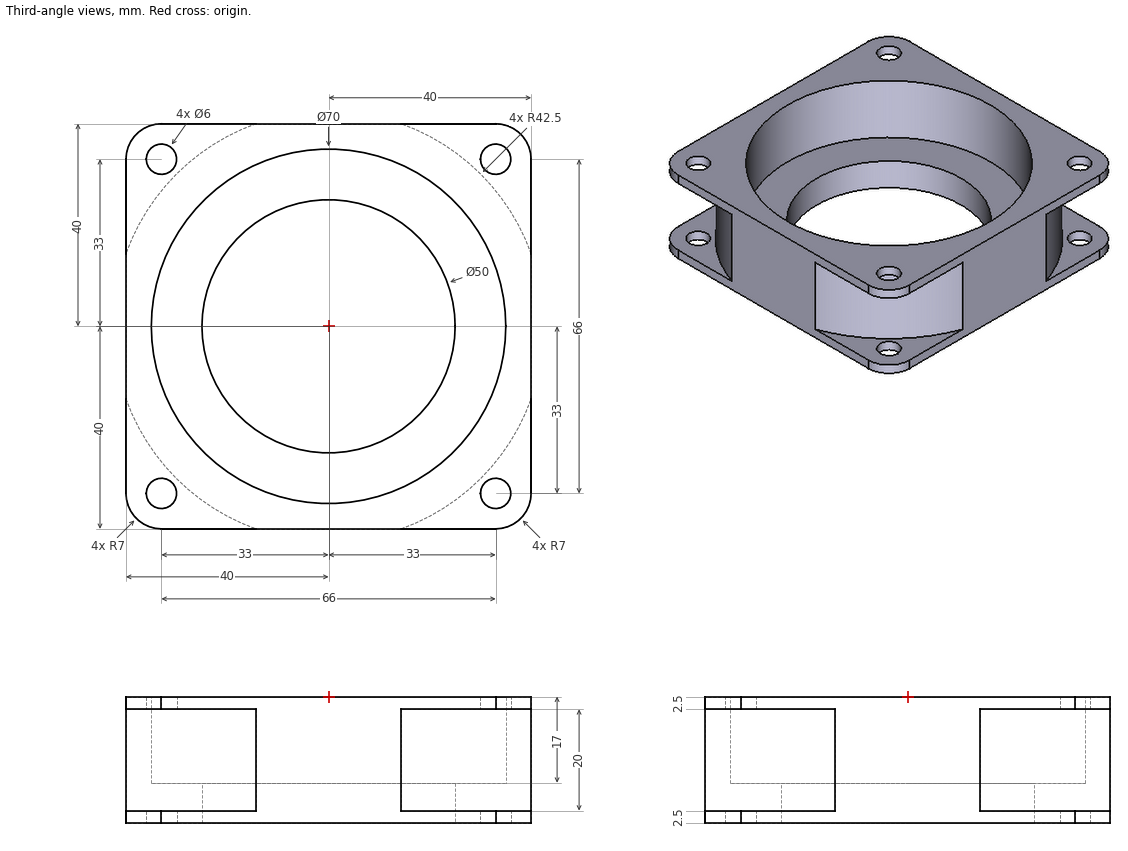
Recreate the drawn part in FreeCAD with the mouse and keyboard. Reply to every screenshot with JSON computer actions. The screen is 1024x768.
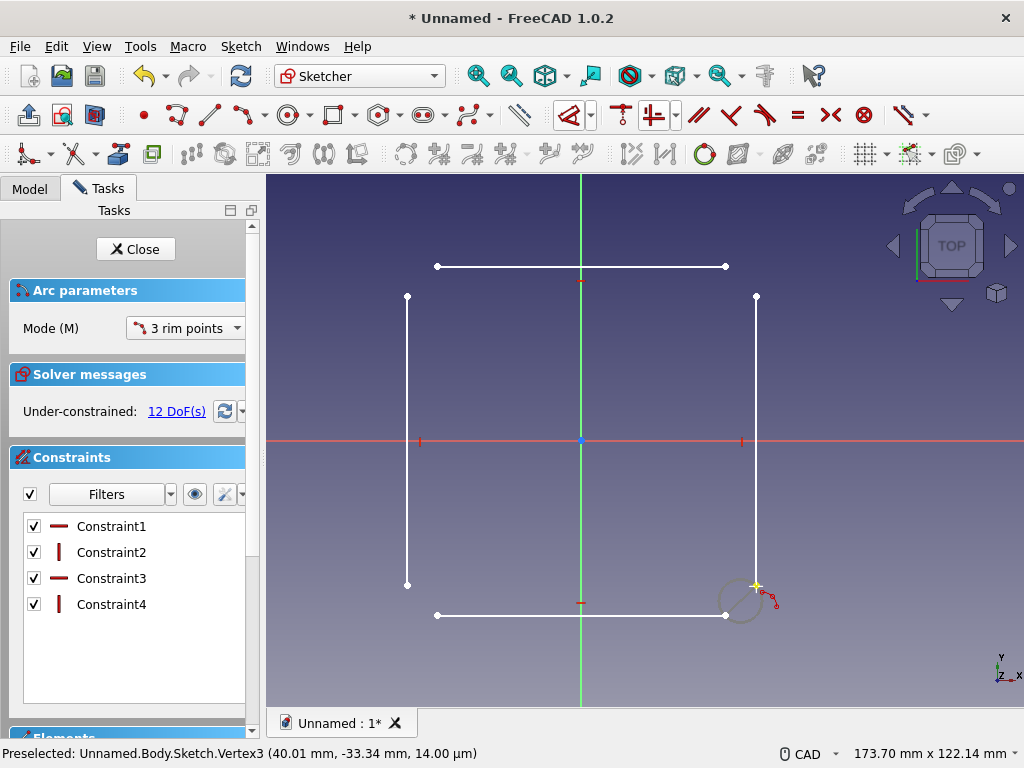
{"action": "scroll", "coordinate": [747, 606], "scroll_direction": "up", "scroll_amount": 3}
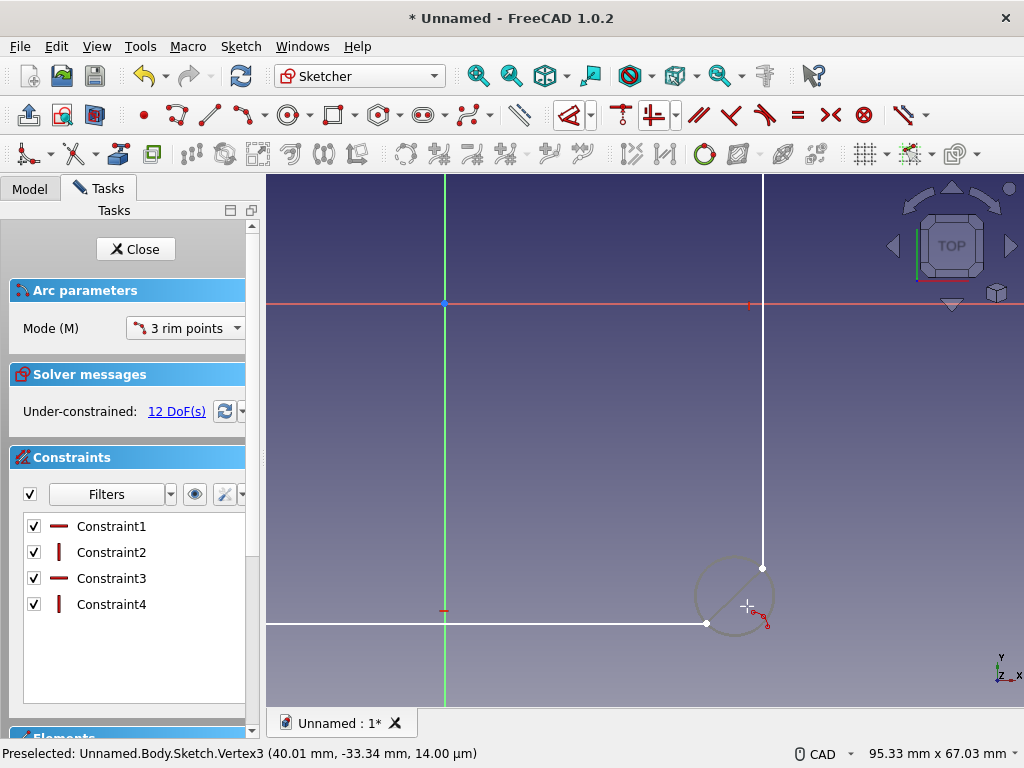
{"action": "left_click", "coordinate": [746, 606]}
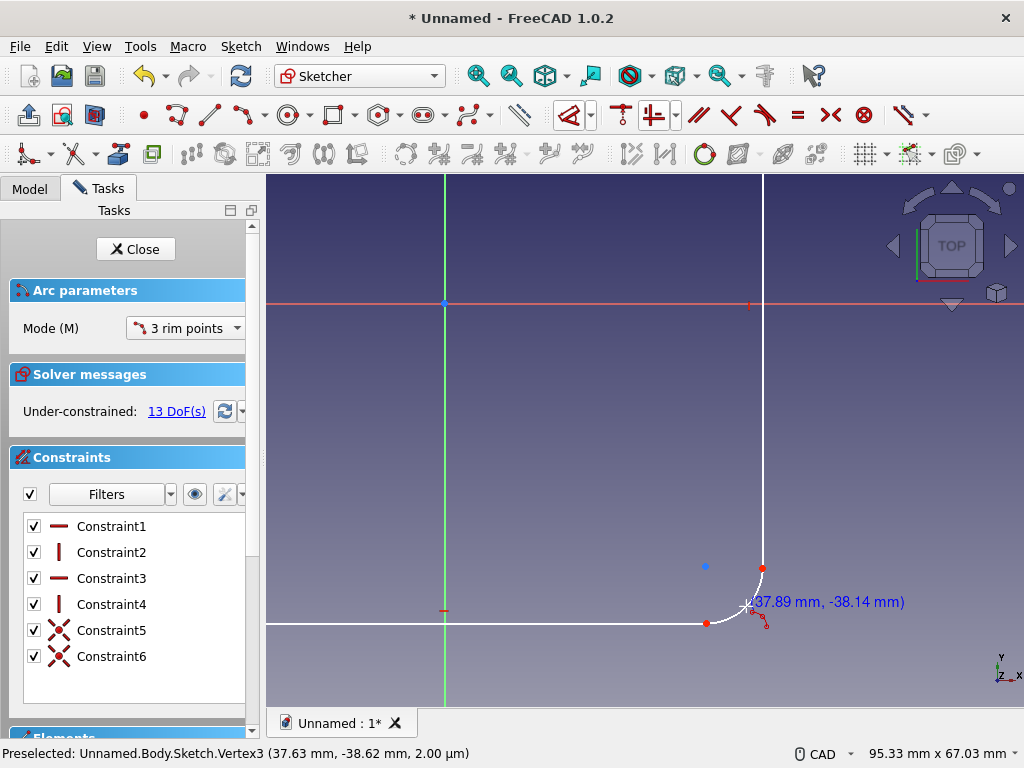
{"action": "scroll", "coordinate": [737, 607], "scroll_direction": "down", "scroll_amount": 3}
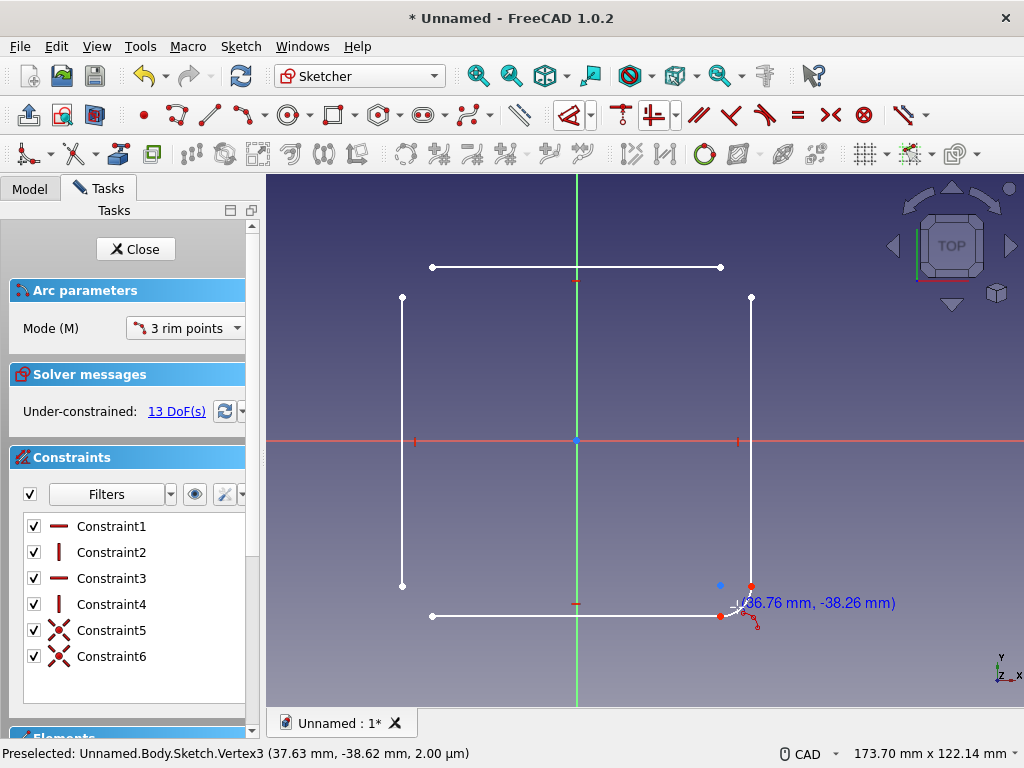
{"action": "left_click", "coordinate": [751, 297]}
{"action": "left_click", "coordinate": [720, 267]}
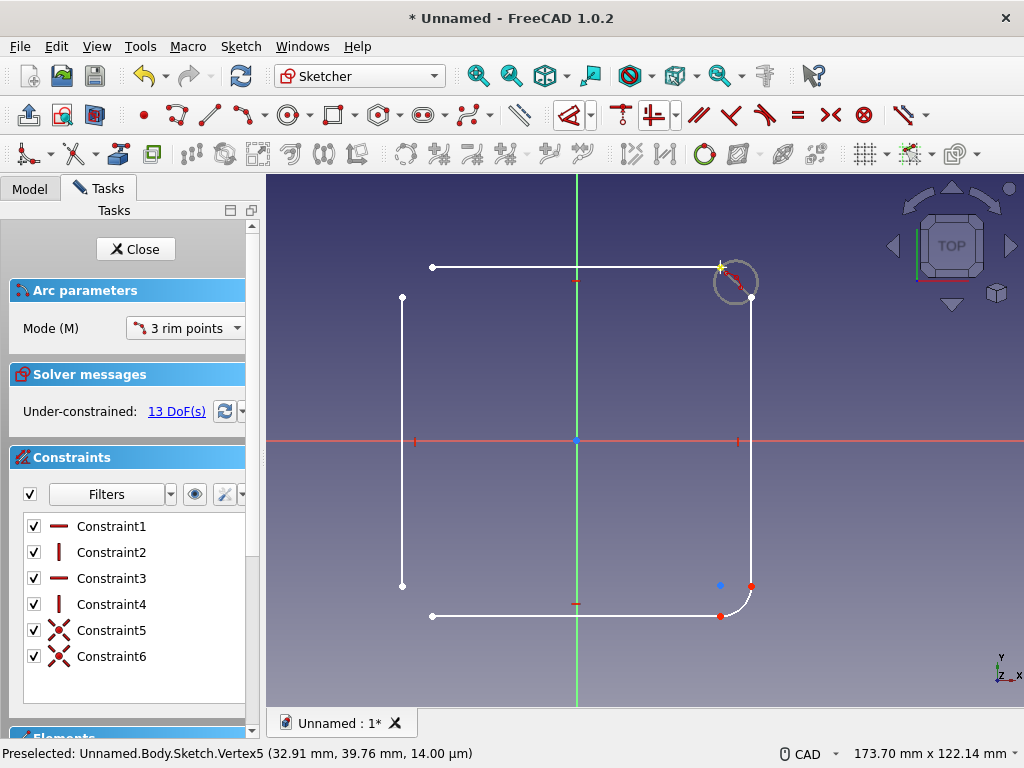
{"action": "scroll", "coordinate": [742, 275], "scroll_direction": "up", "scroll_amount": 3}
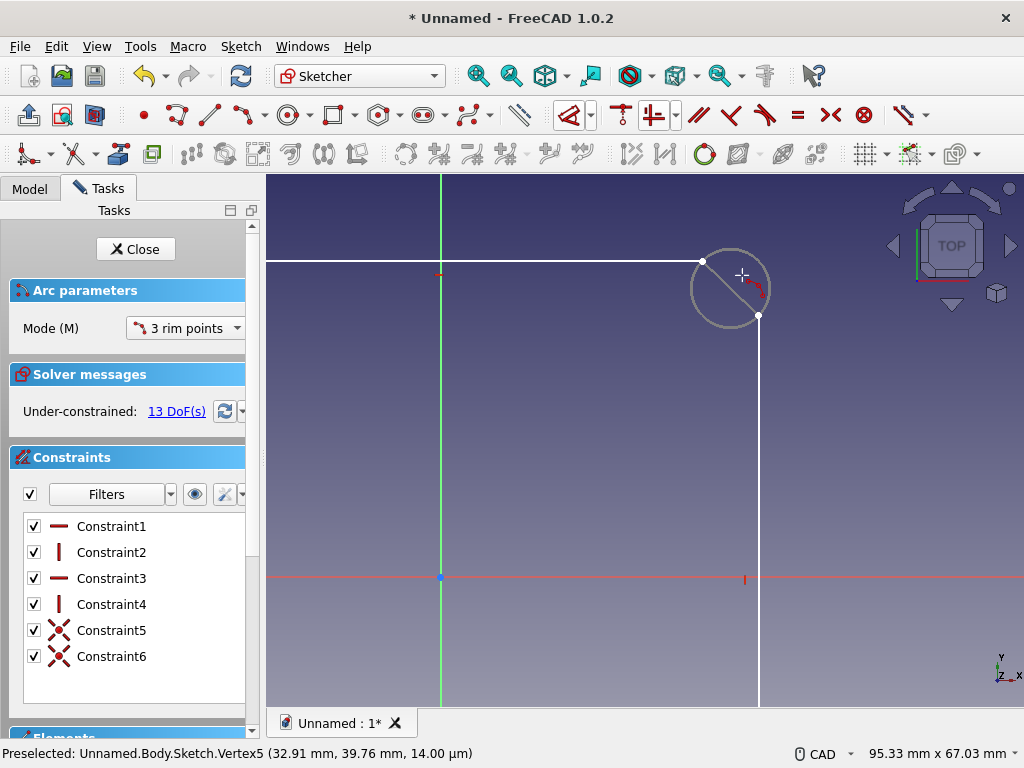
{"action": "left_click", "coordinate": [742, 275]}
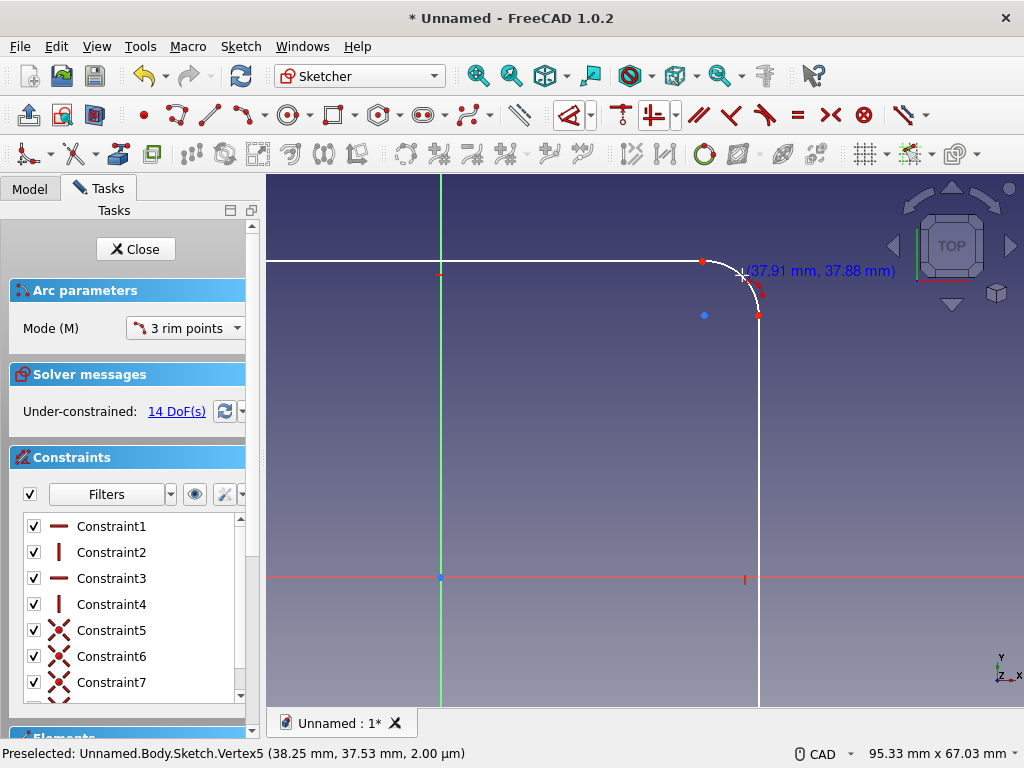
{"action": "scroll", "coordinate": [742, 274], "scroll_direction": "down", "scroll_amount": 3}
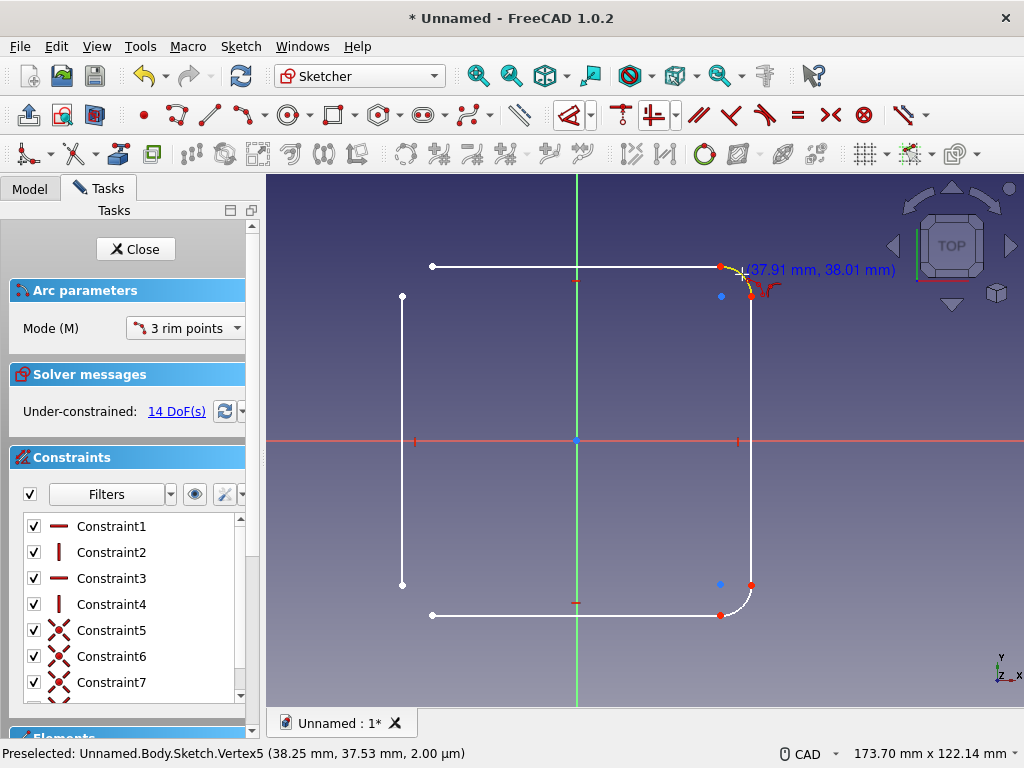
{"action": "left_click", "coordinate": [432, 267]}
{"action": "left_click", "coordinate": [402, 297]}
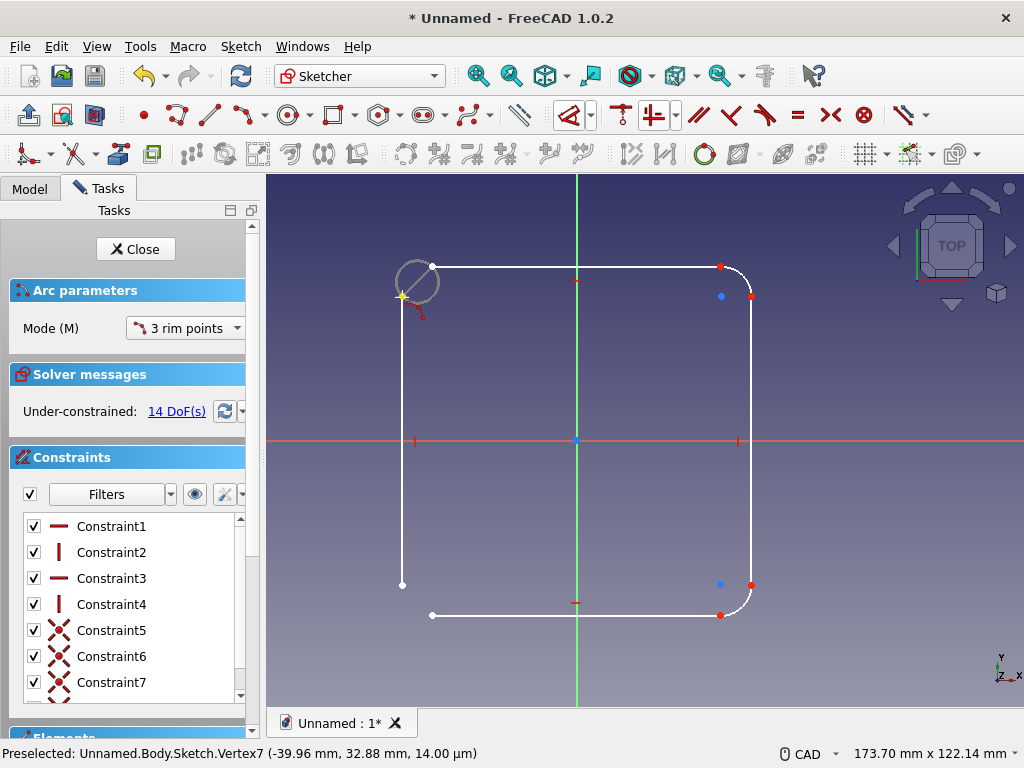
{"action": "scroll", "coordinate": [411, 275], "scroll_direction": "up", "scroll_amount": 3}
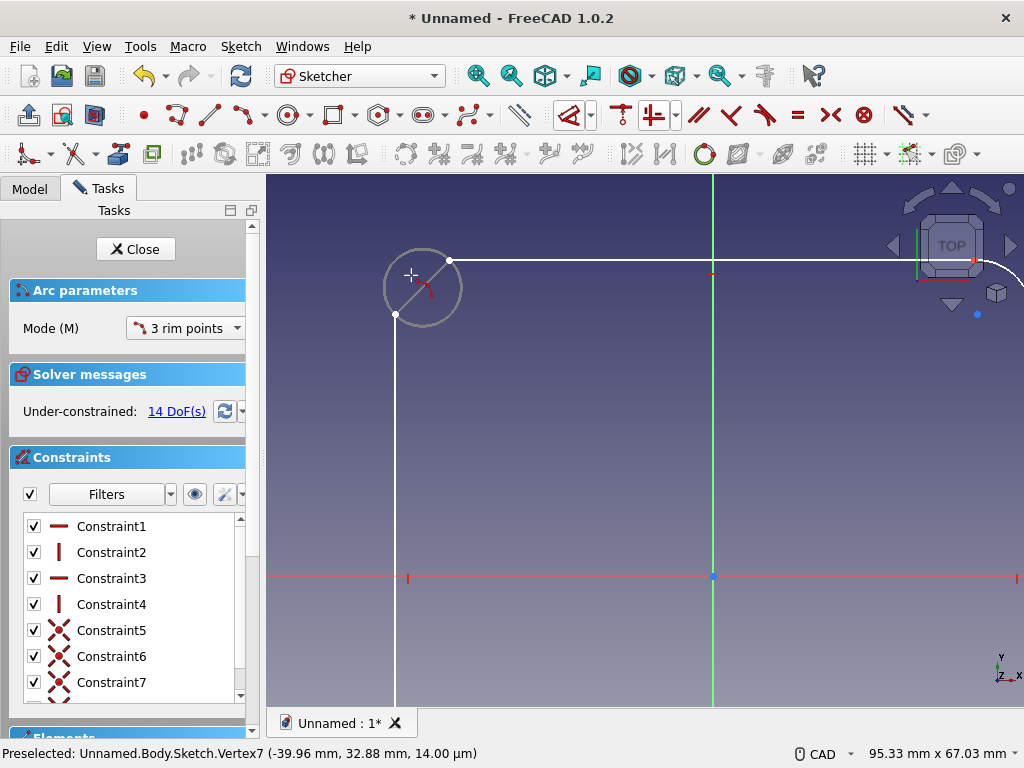
{"action": "left_click", "coordinate": [411, 275]}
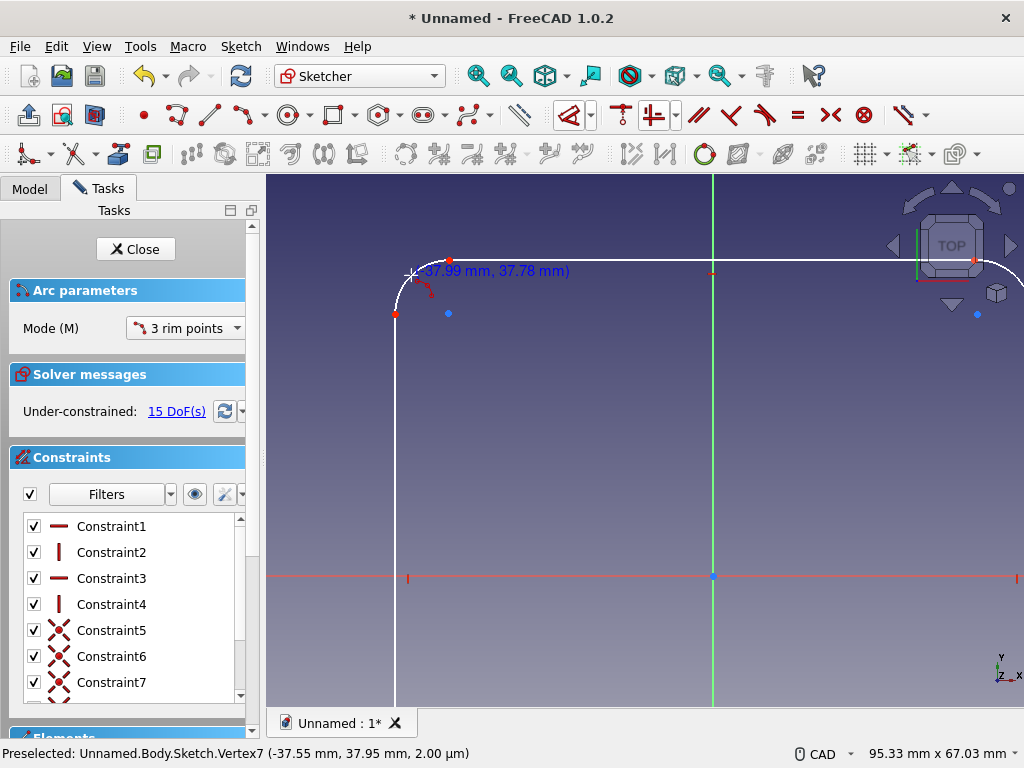
{"action": "scroll", "coordinate": [410, 275], "scroll_direction": "down", "scroll_amount": 3}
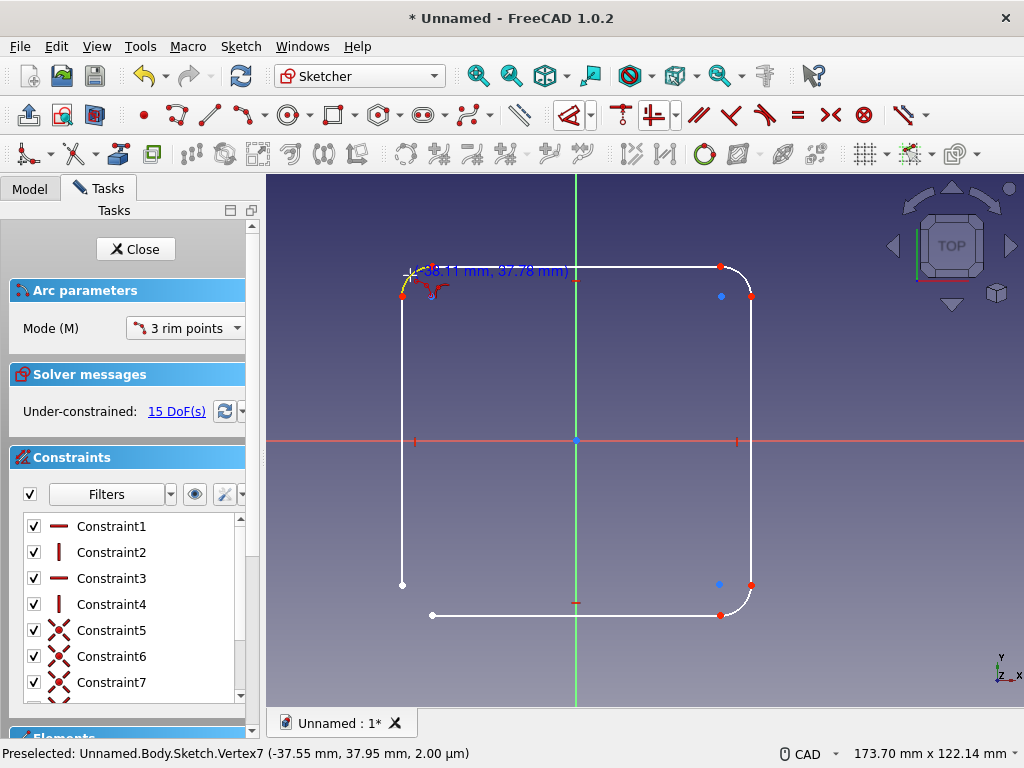
{"action": "left_click", "coordinate": [402, 586]}
{"action": "left_click", "coordinate": [432, 616]}